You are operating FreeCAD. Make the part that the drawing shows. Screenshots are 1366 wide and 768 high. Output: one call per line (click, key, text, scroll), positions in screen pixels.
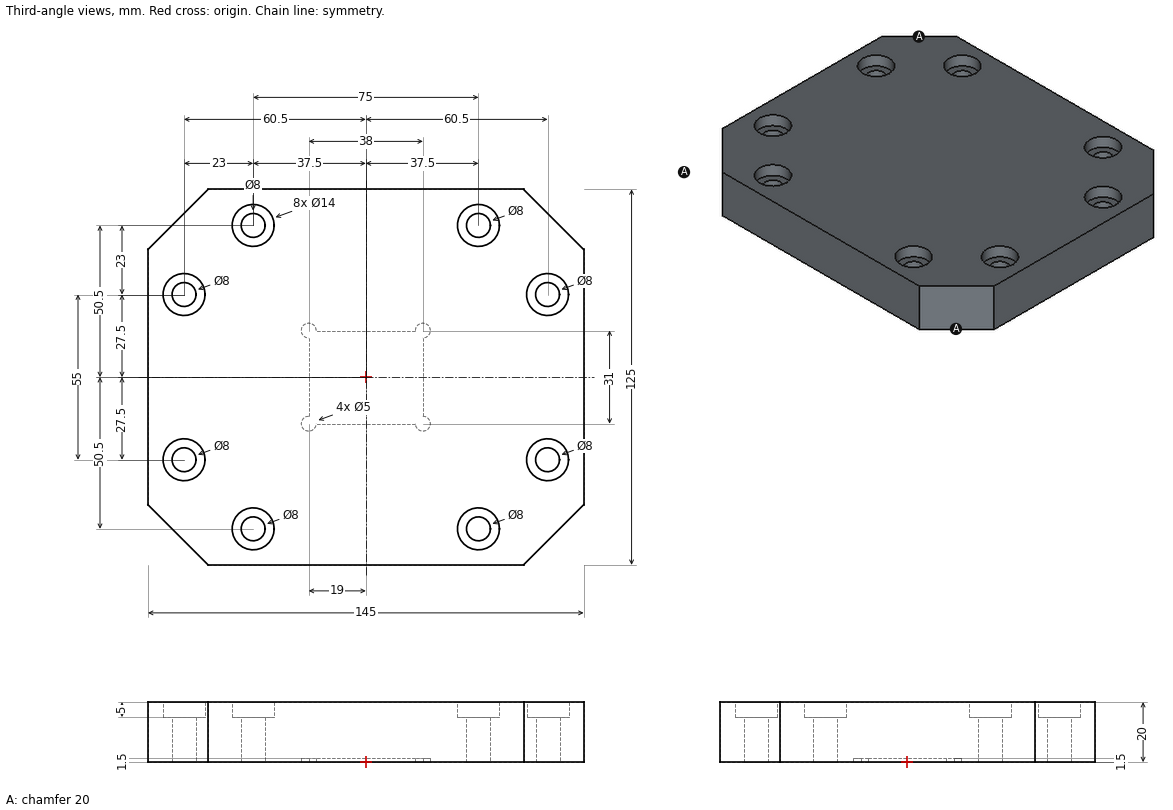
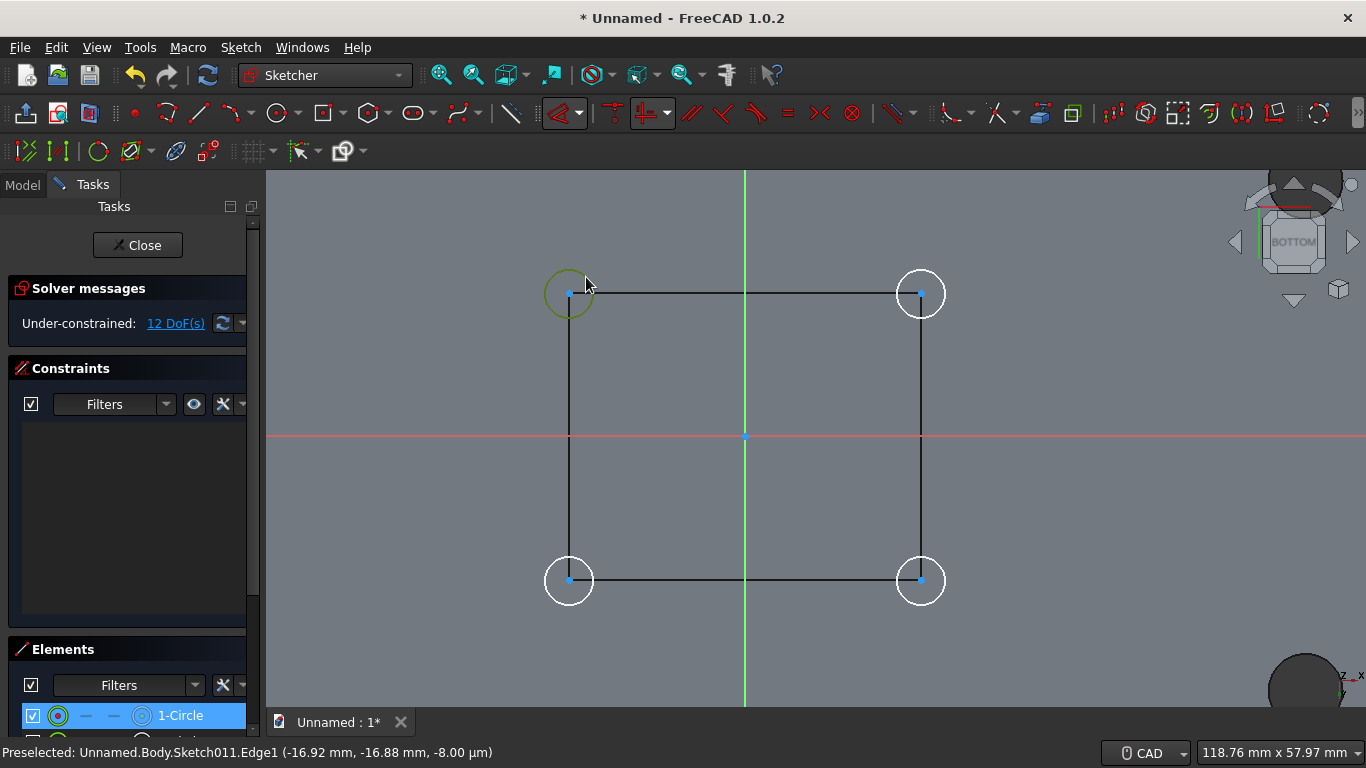
click(938, 277)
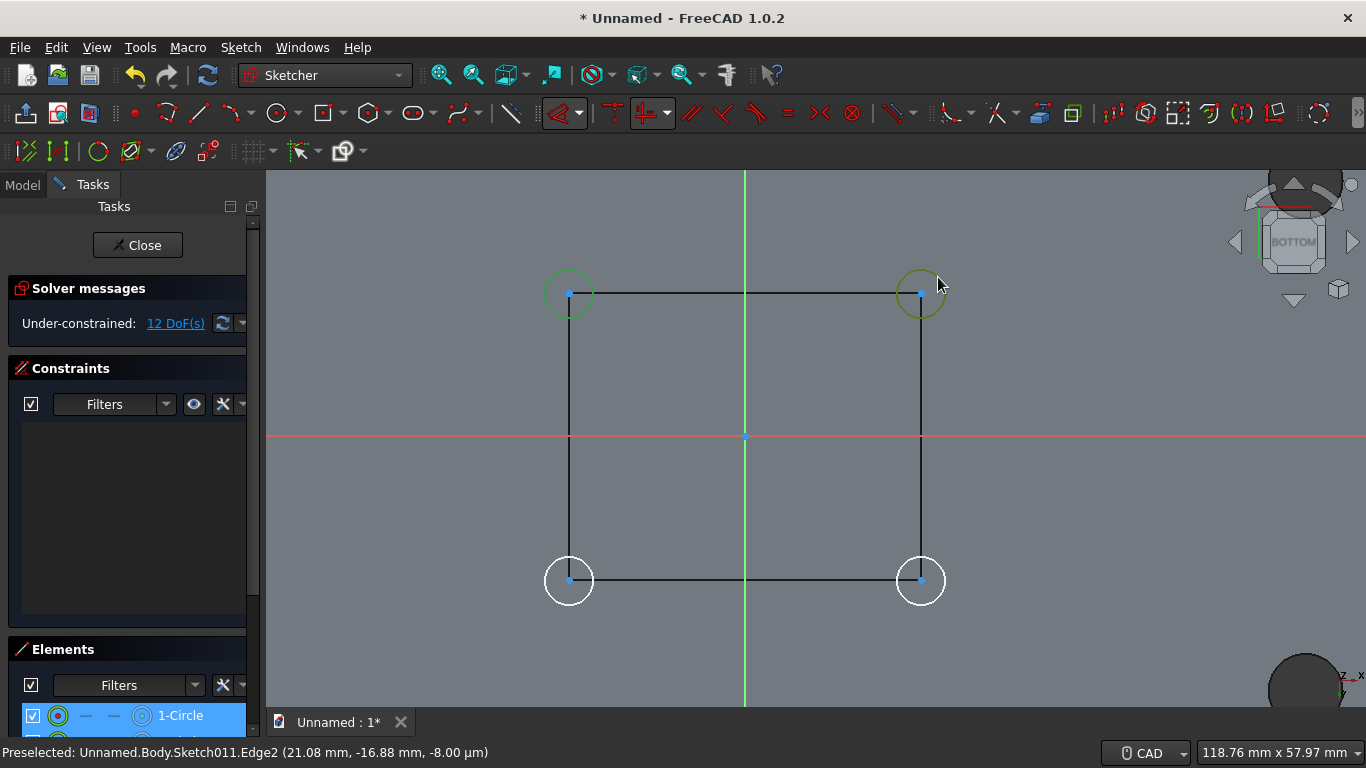
click(938, 564)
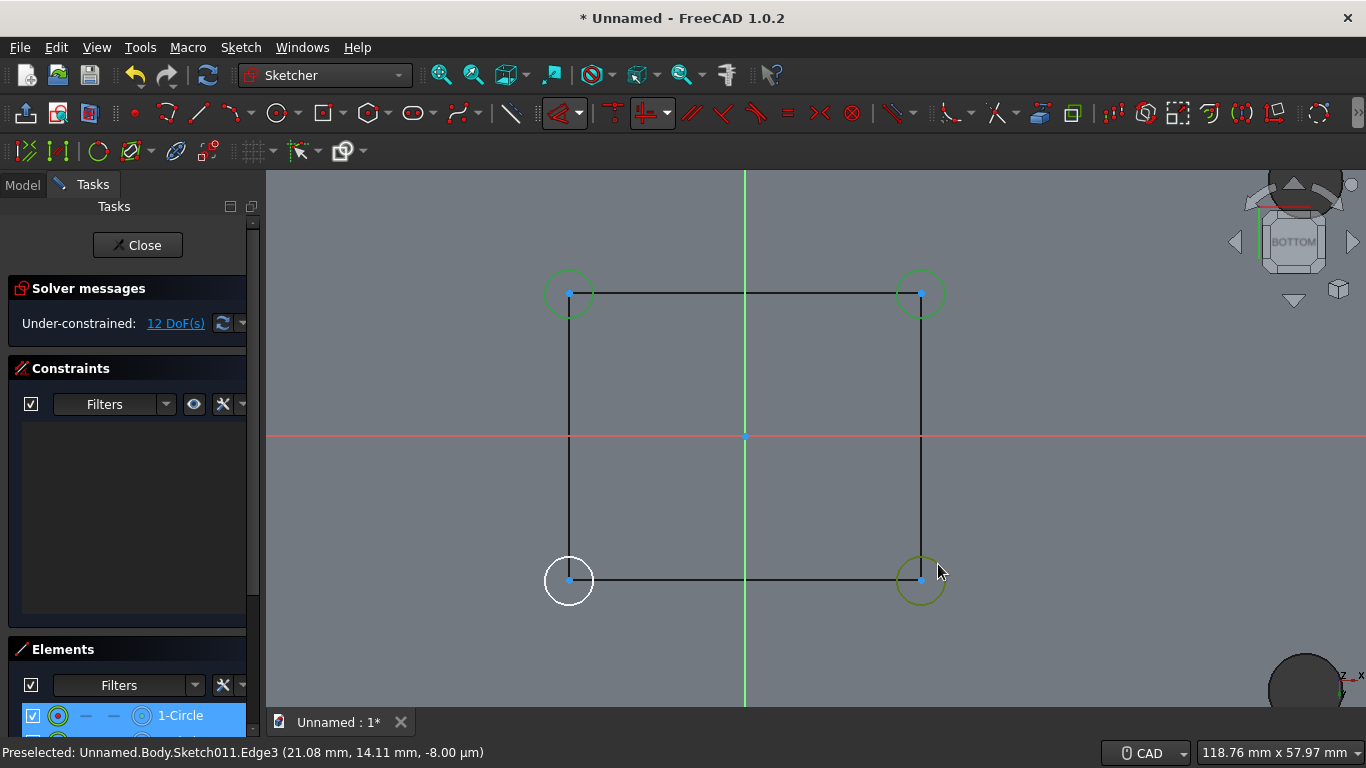
click(586, 564)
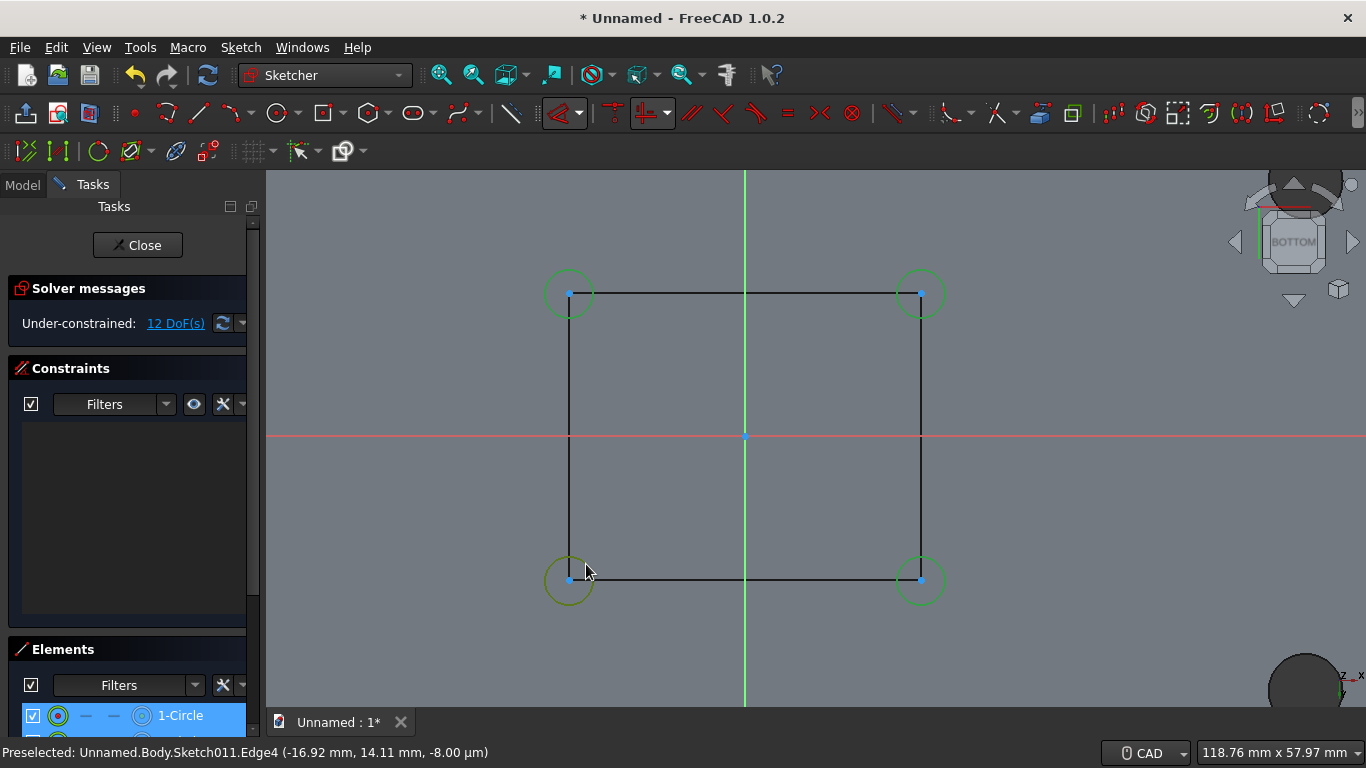
click(788, 114)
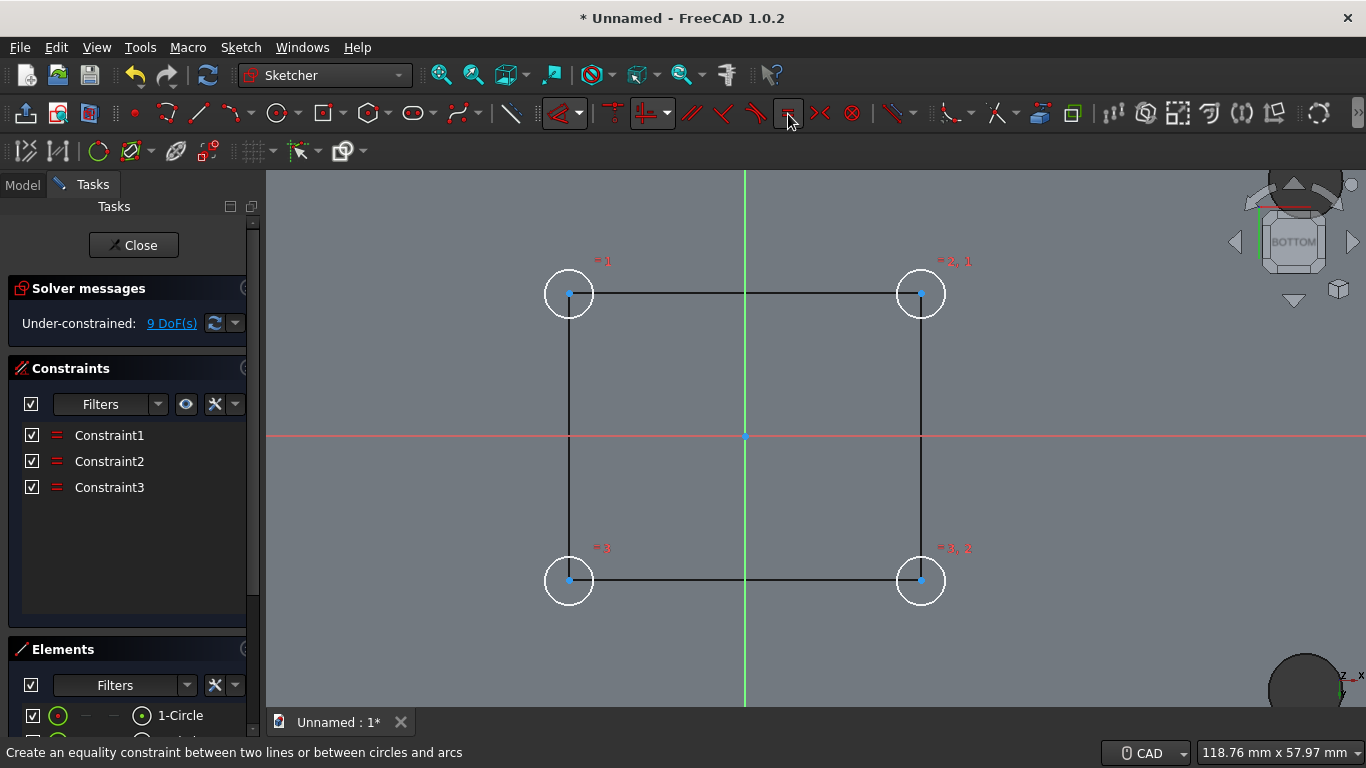
click(569, 294)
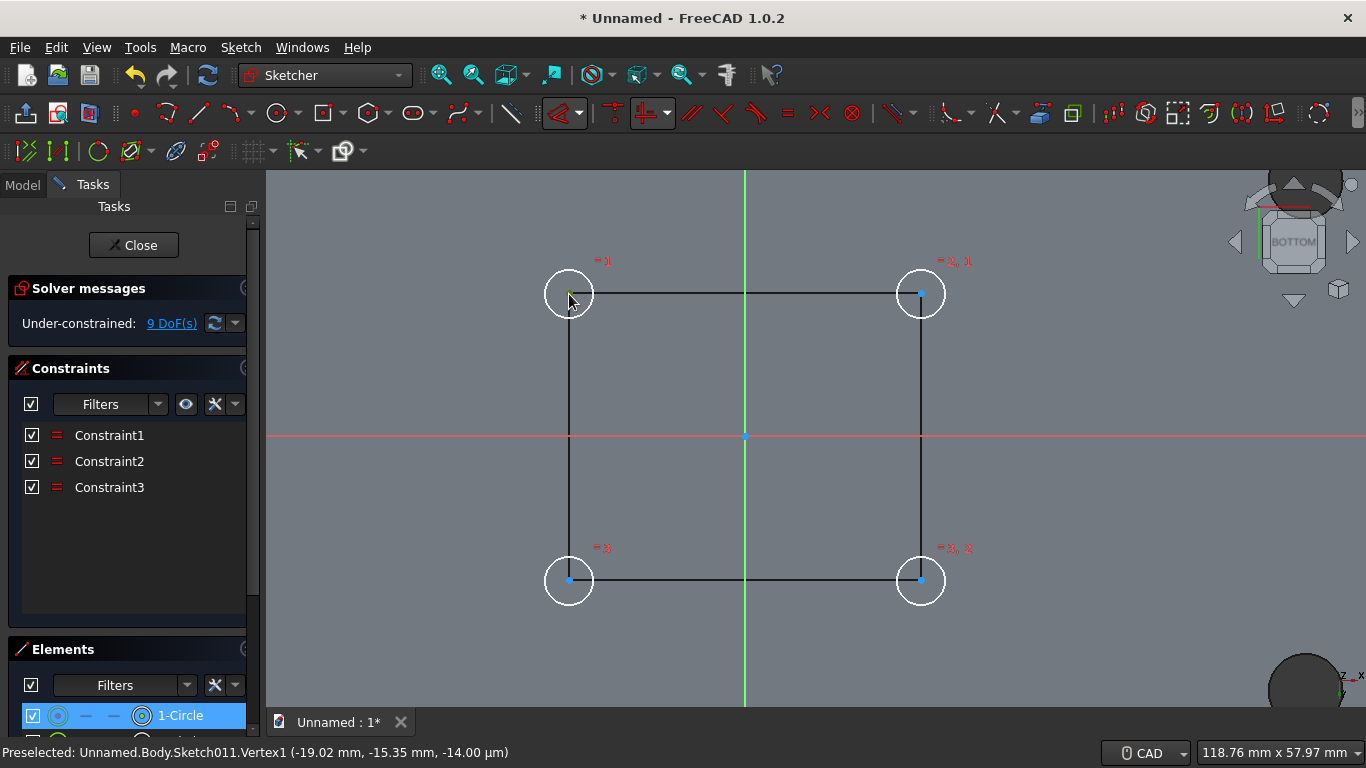
click(921, 294)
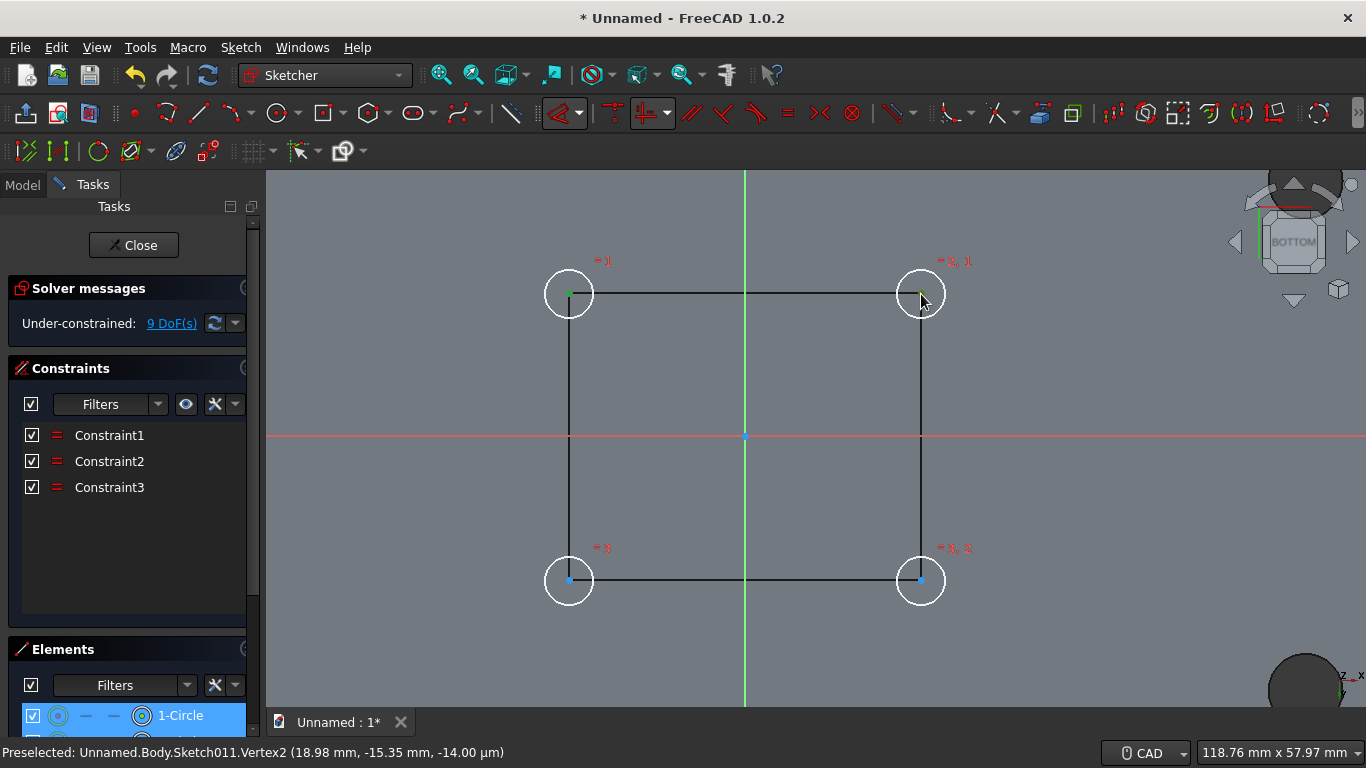
click(745, 645)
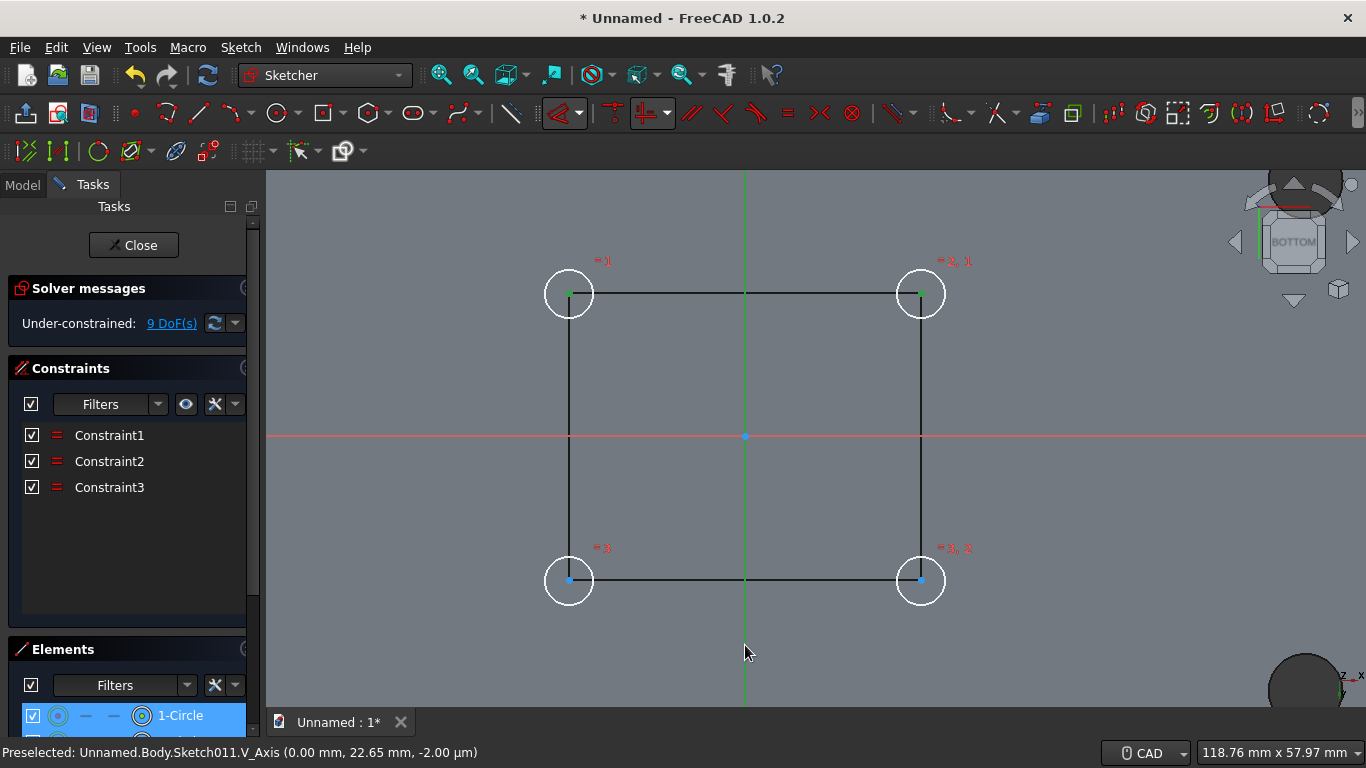
click(820, 114)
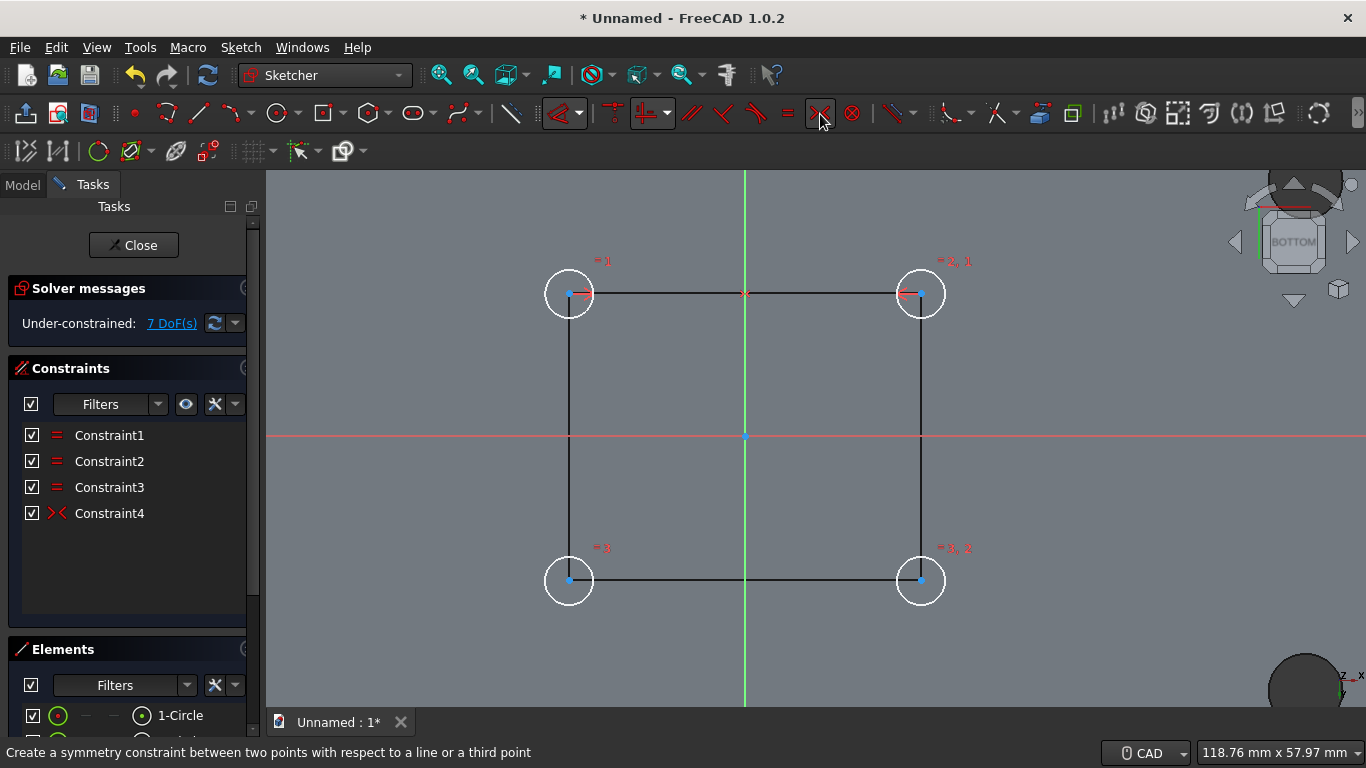
click(921, 294)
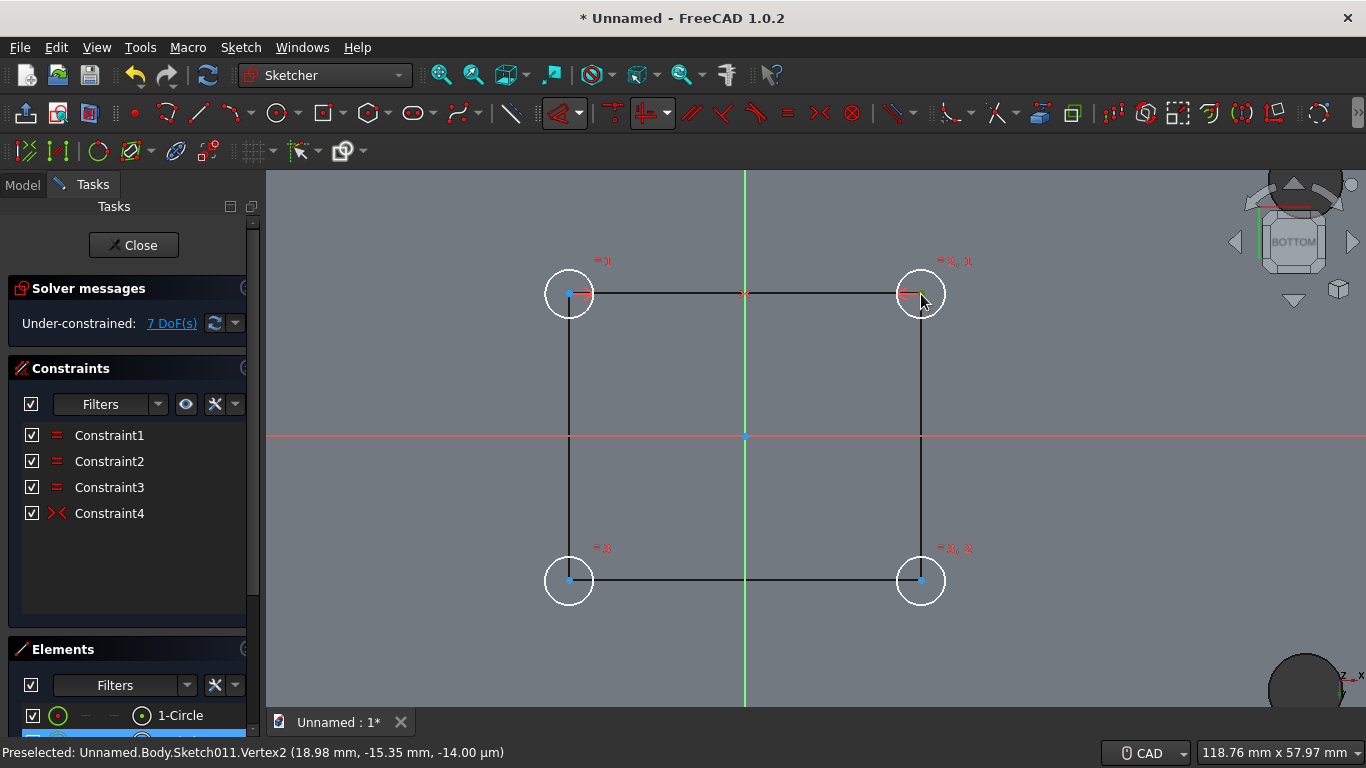
click(921, 581)